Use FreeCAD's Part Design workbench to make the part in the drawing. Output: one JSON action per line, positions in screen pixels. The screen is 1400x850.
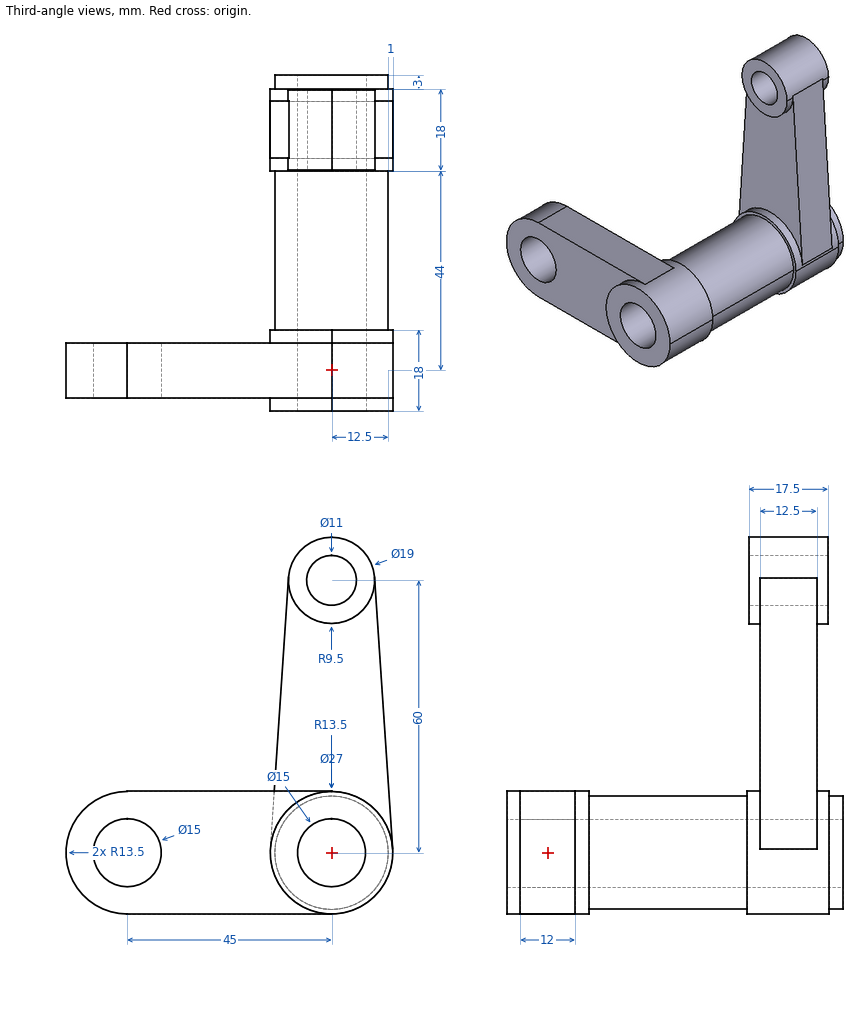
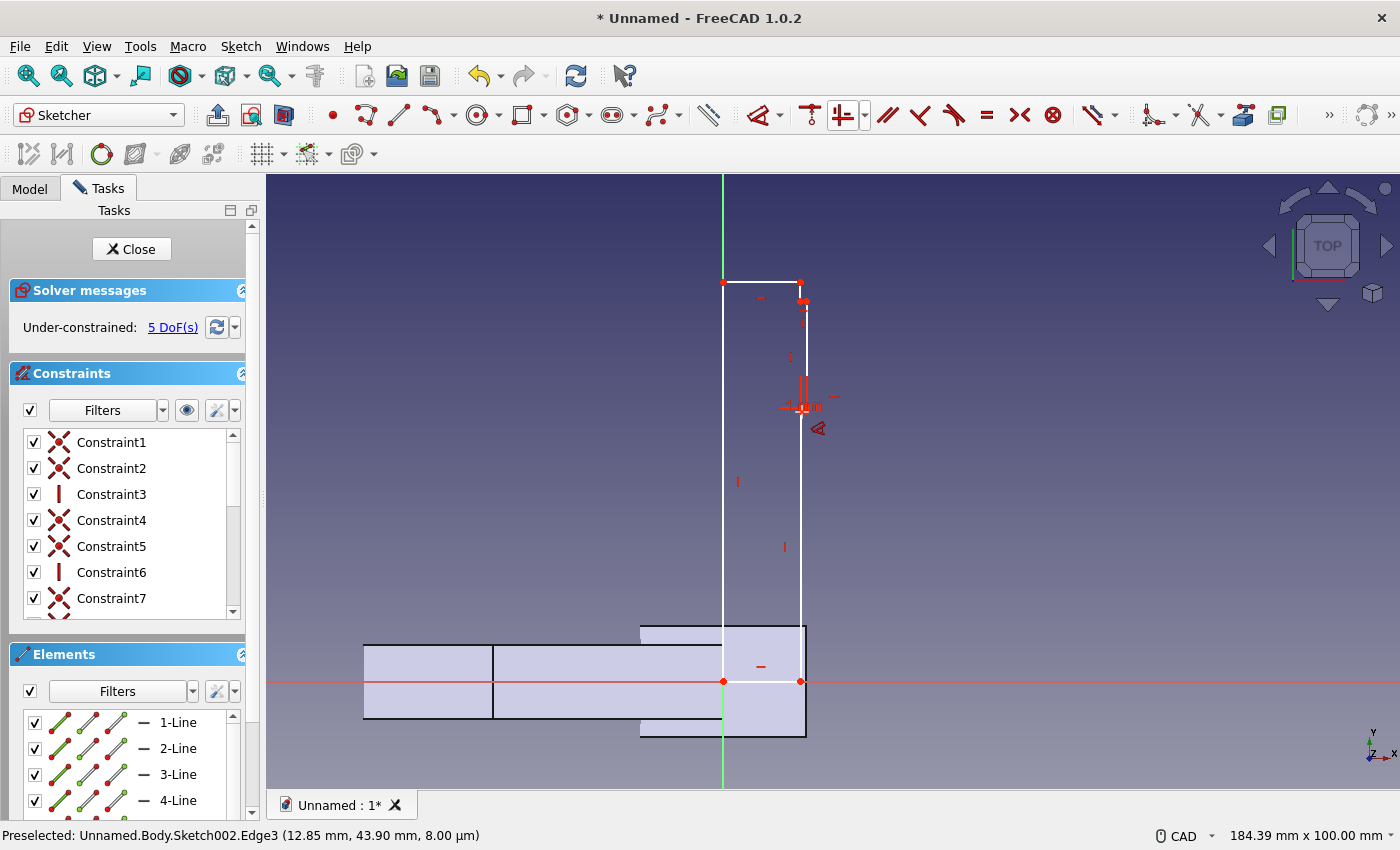
{"action": "scroll", "coordinate": [805, 301], "scroll_direction": "up", "scroll_amount": 10}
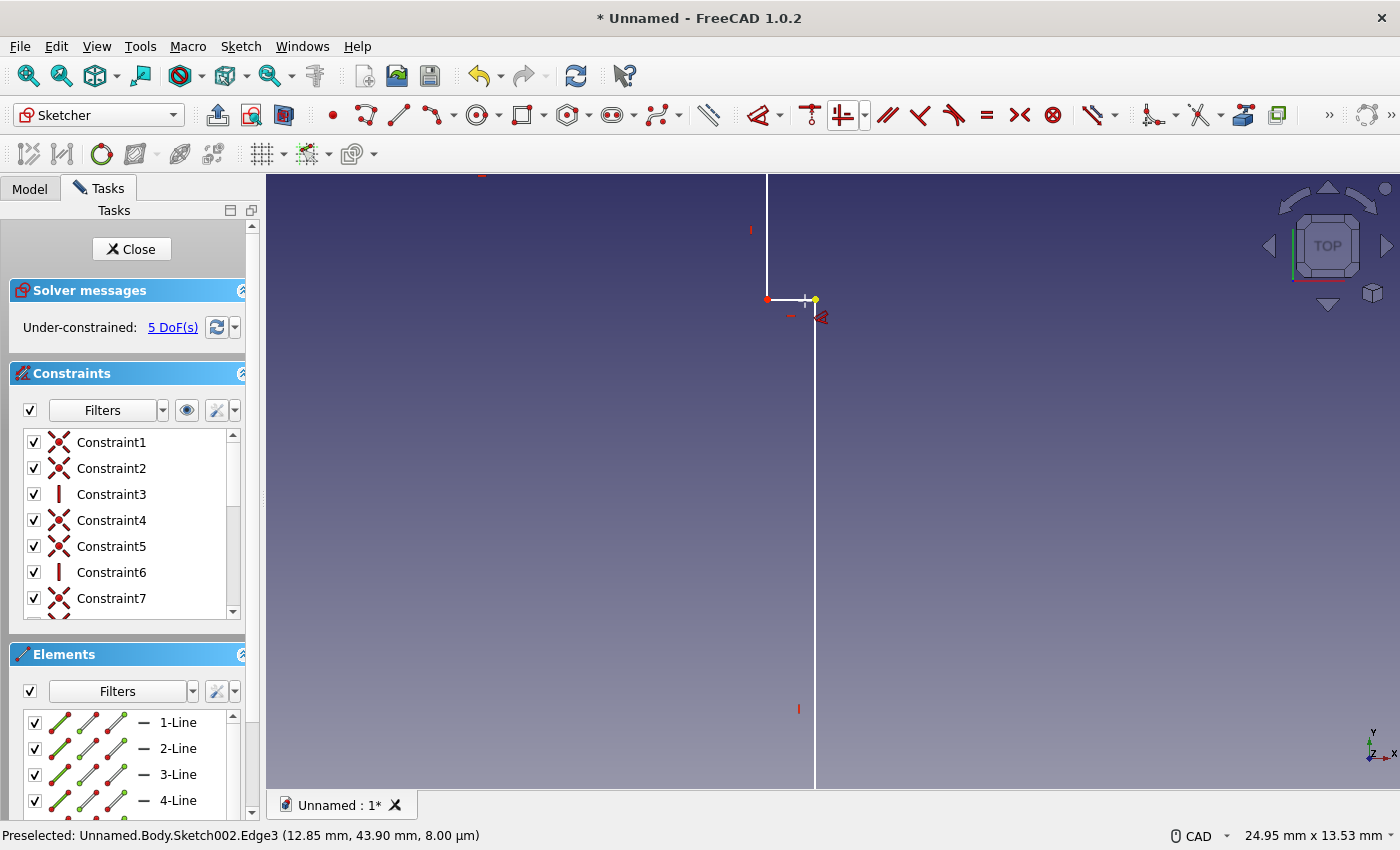
{"action": "left_click", "coordinate": [801, 300]}
{"action": "left_click", "coordinate": [791, 266]}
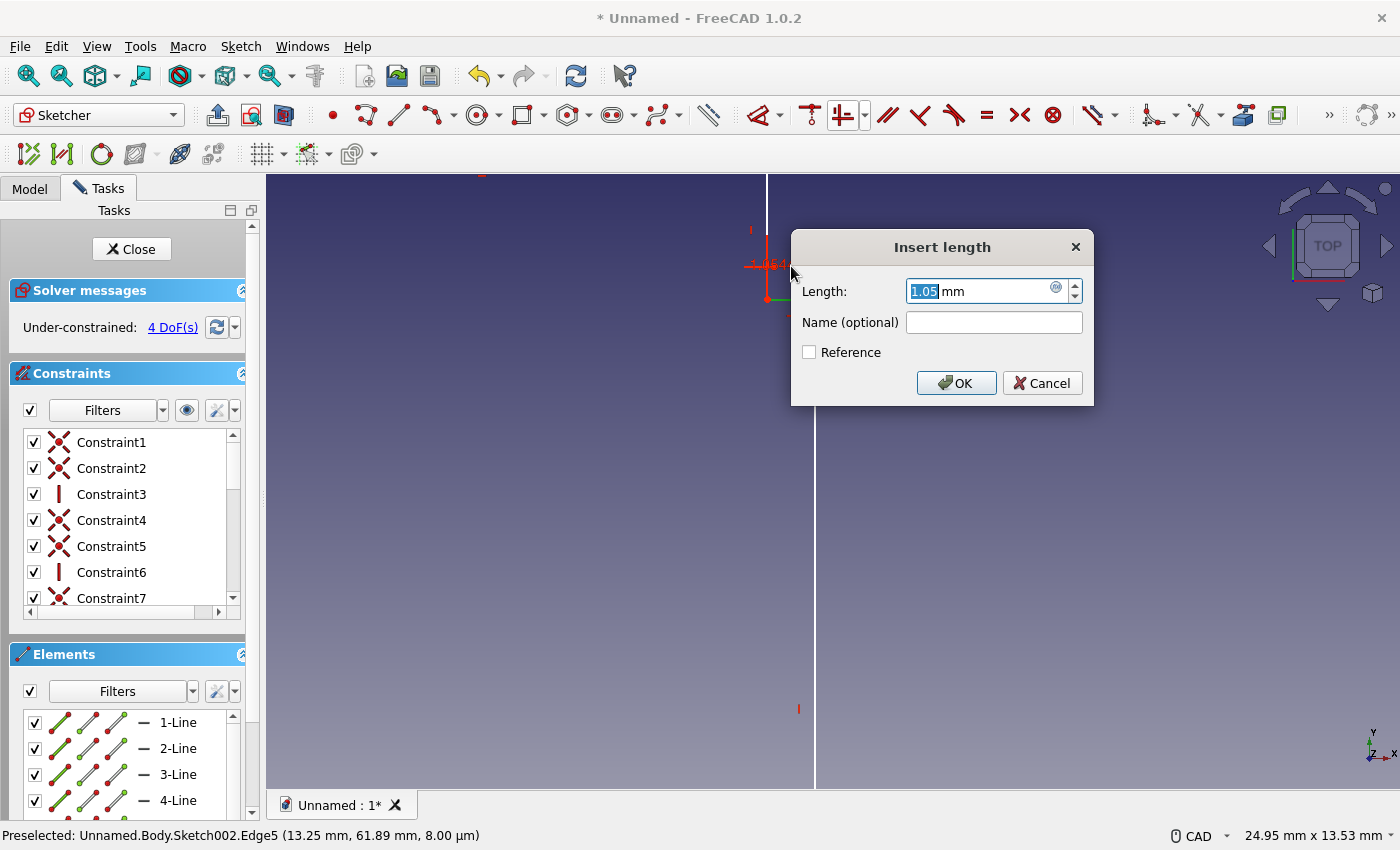
{"action": "type", "text": "1"}
{"action": "key", "text": "Return"}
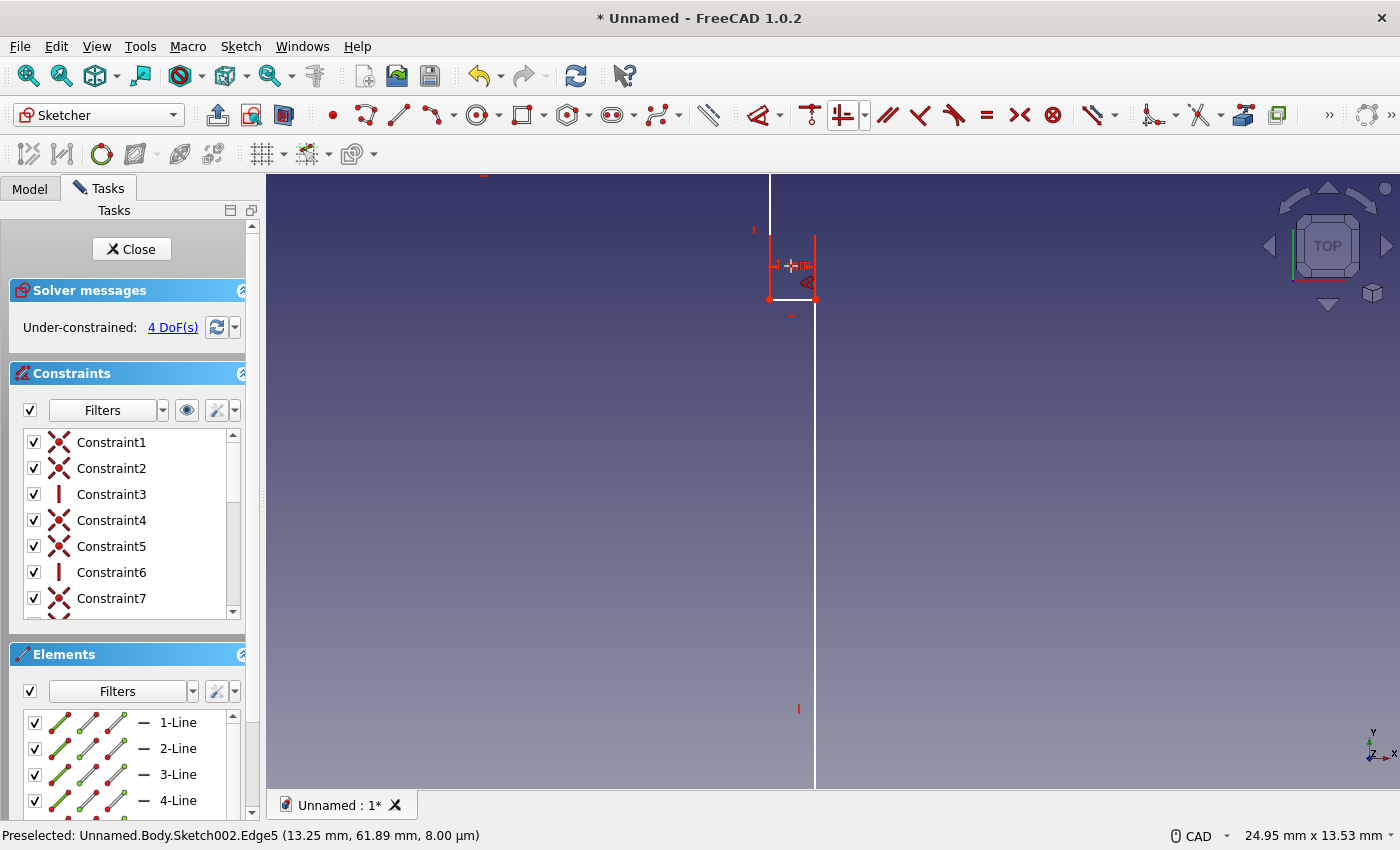
{"action": "scroll", "coordinate": [805, 301], "scroll_direction": "down", "scroll_amount": 10}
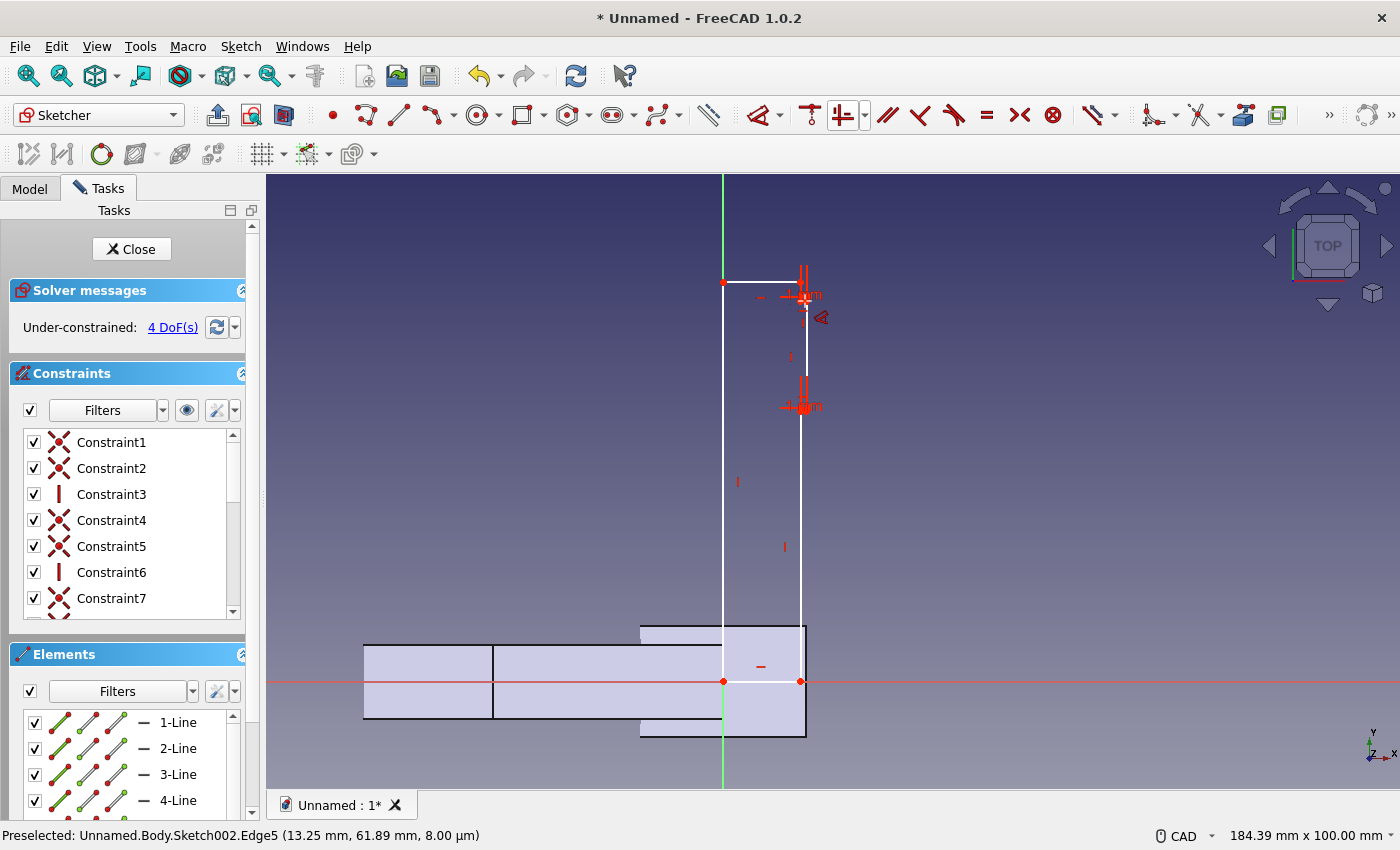
{"action": "scroll", "coordinate": [801, 295], "scroll_direction": "up", "scroll_amount": 5}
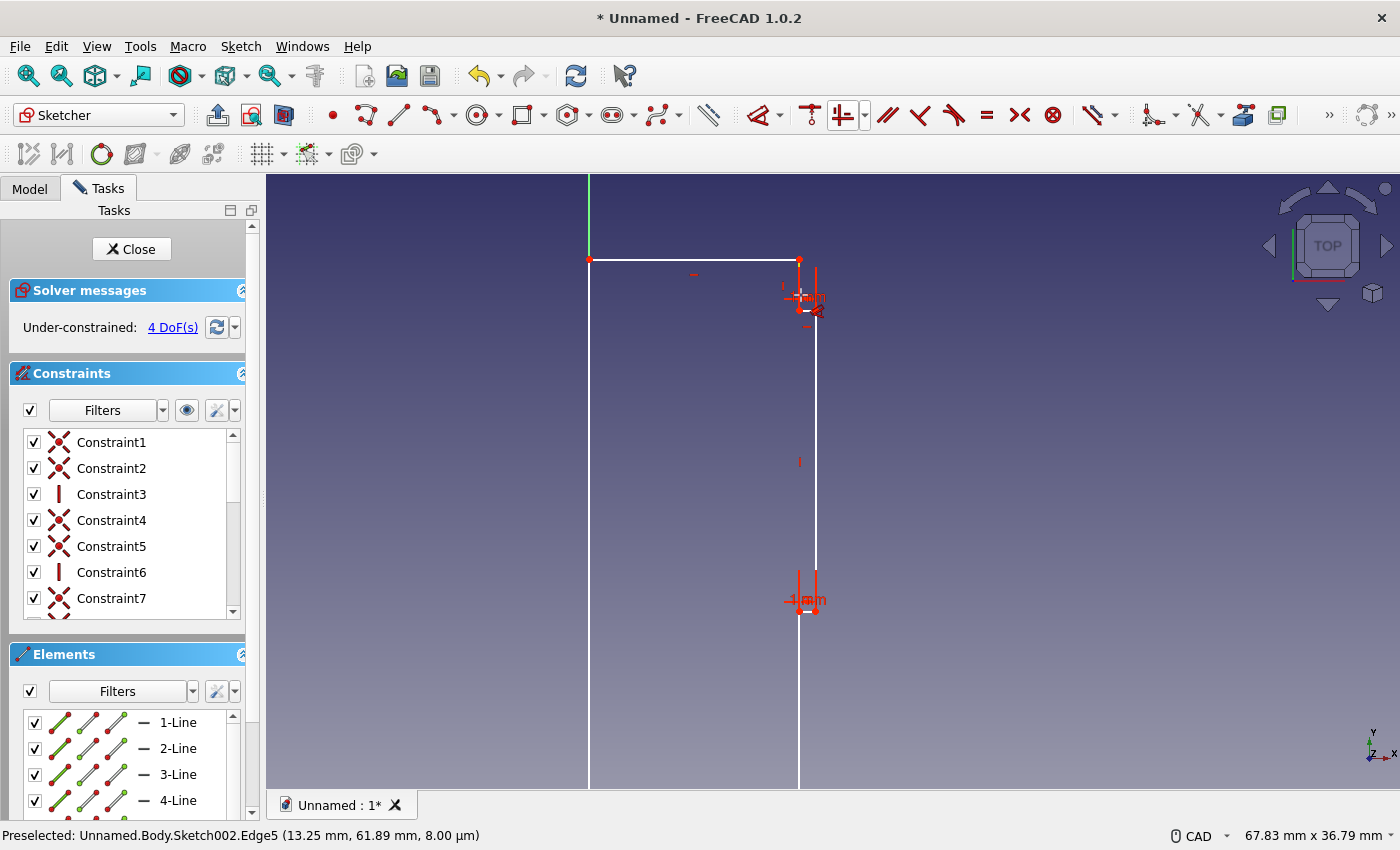
{"action": "left_click", "coordinate": [799, 296]}
{"action": "left_click", "coordinate": [833, 273]}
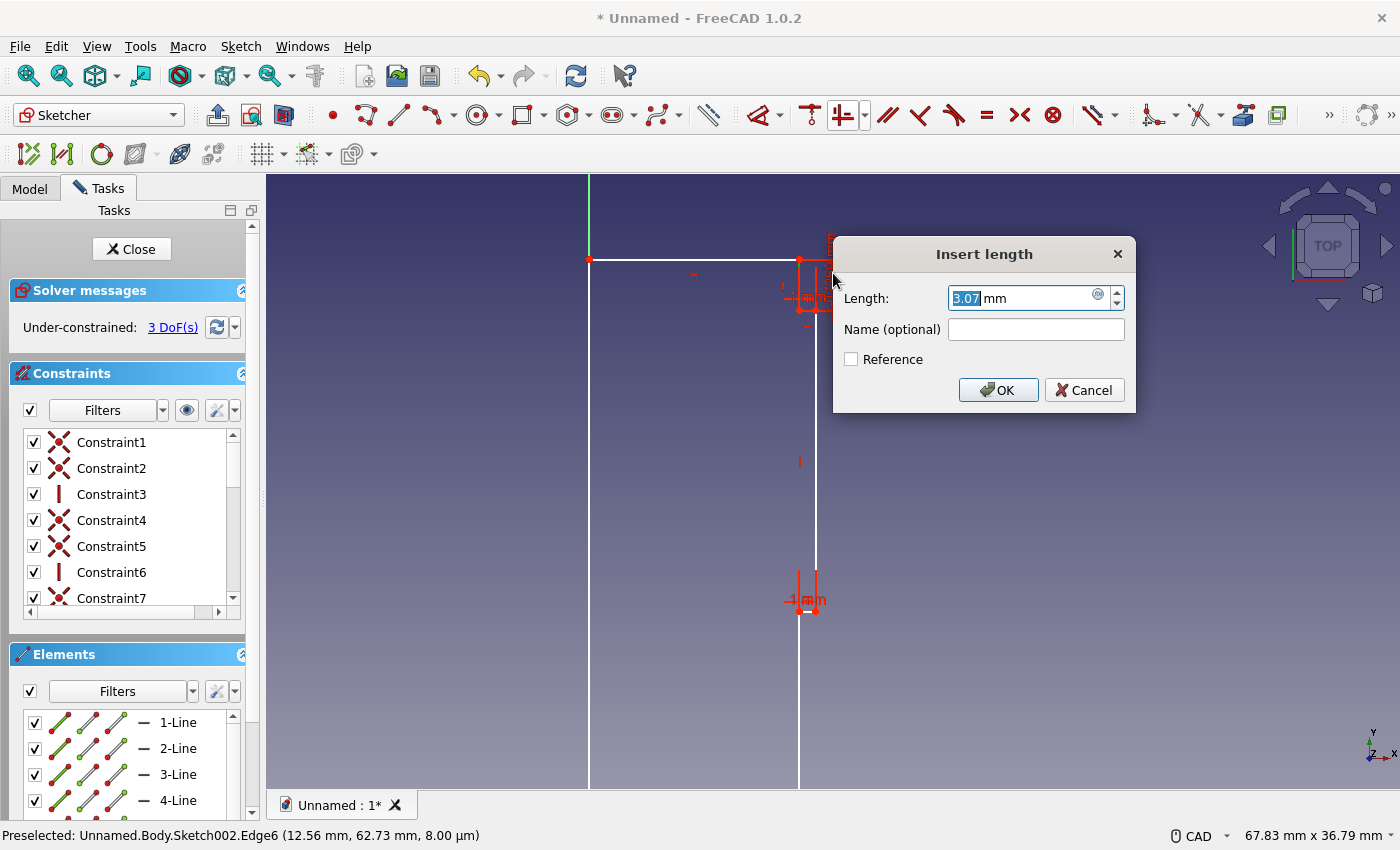
{"action": "type", "text": "3"}
{"action": "key", "text": "Return"}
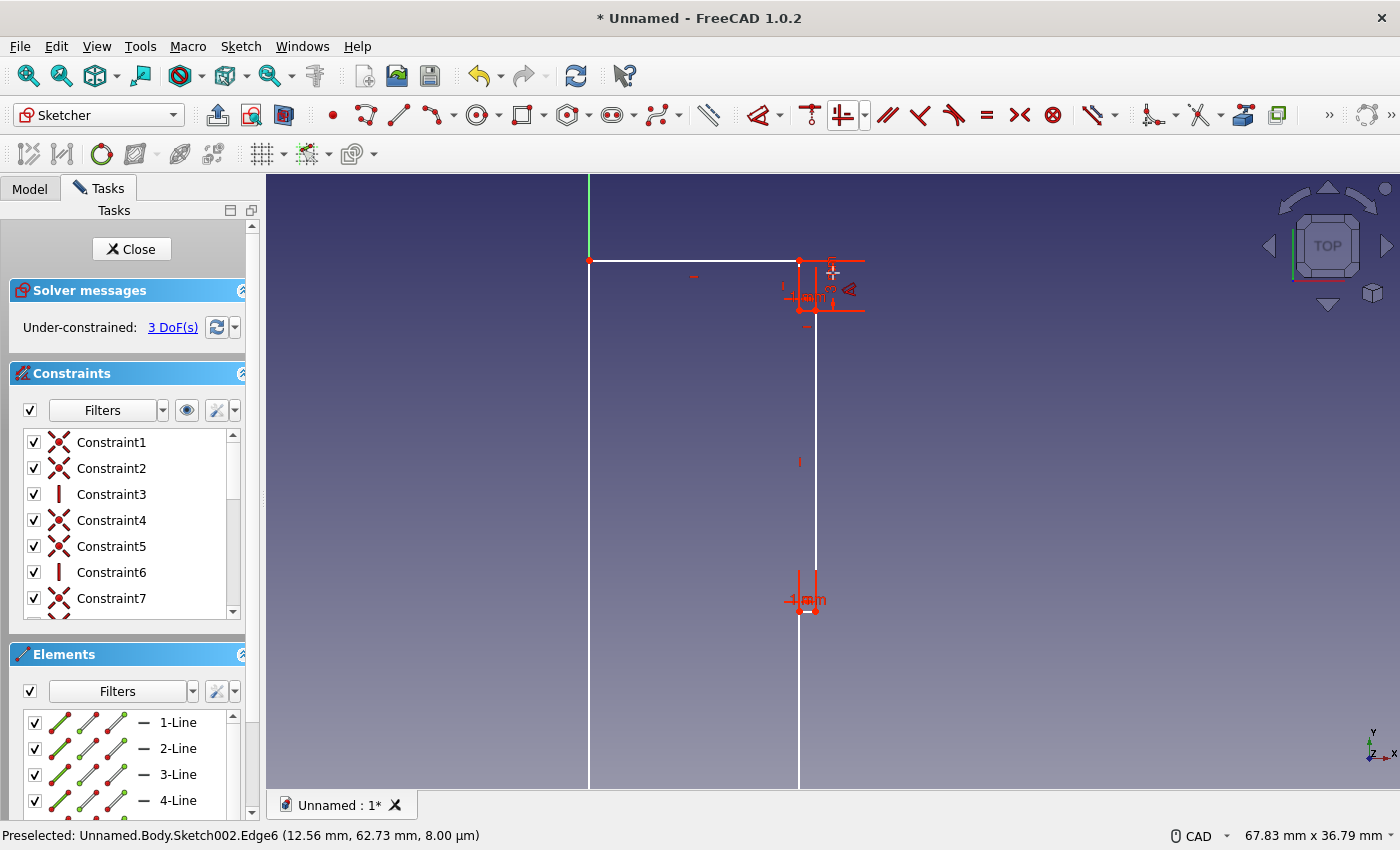
{"action": "left_click", "coordinate": [799, 758]}
{"action": "left_click", "coordinate": [833, 686]}